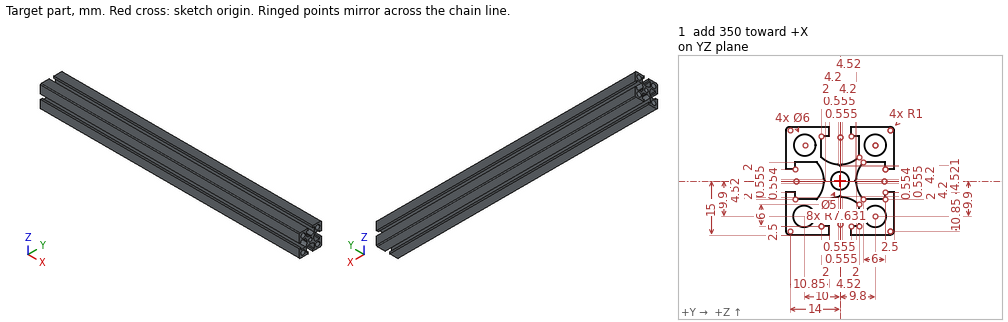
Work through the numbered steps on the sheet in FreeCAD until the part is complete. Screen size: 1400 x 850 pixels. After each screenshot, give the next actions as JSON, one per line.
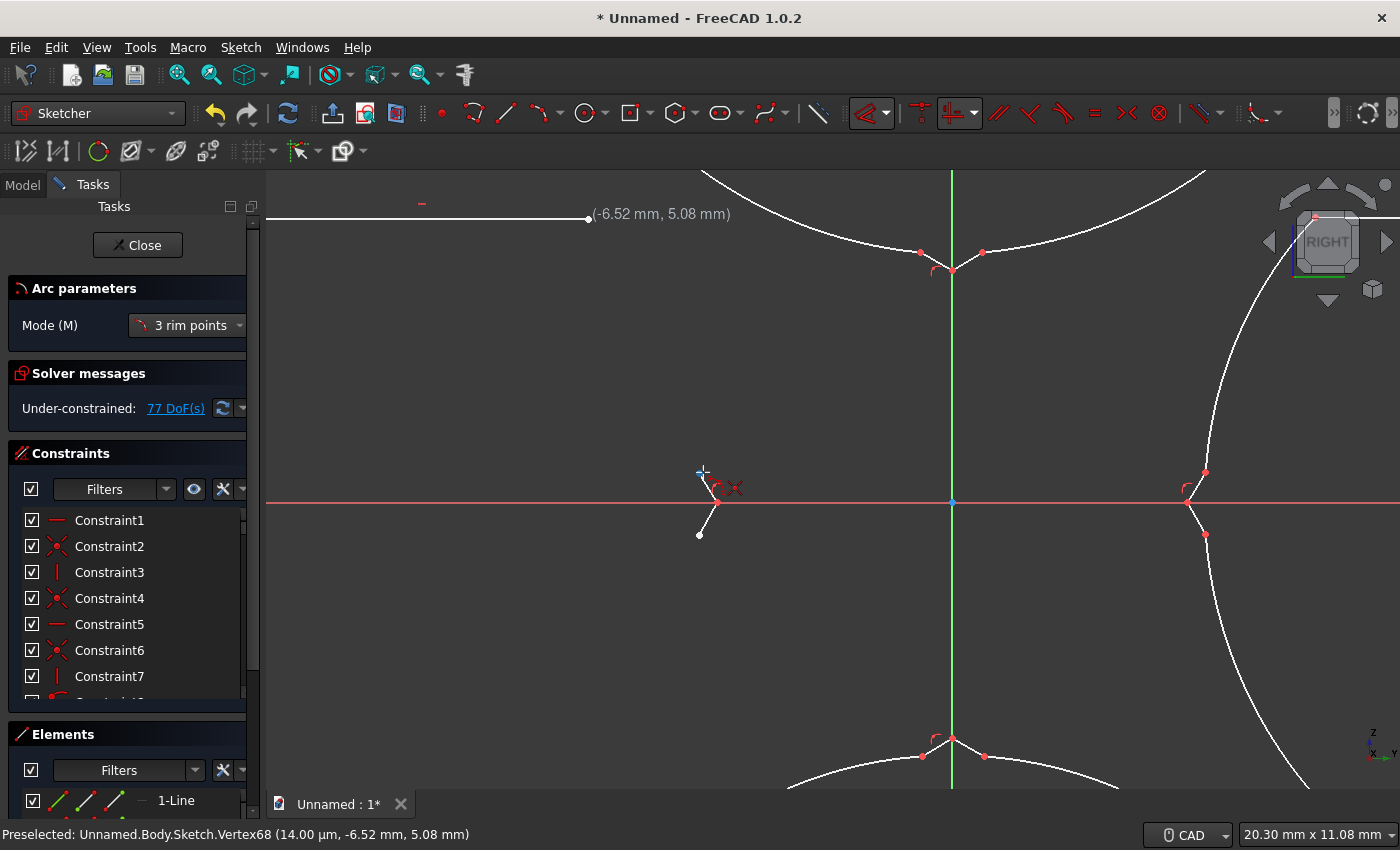
{"action": "left_click", "coordinate": [699, 473]}
{"action": "left_click", "coordinate": [666, 334]}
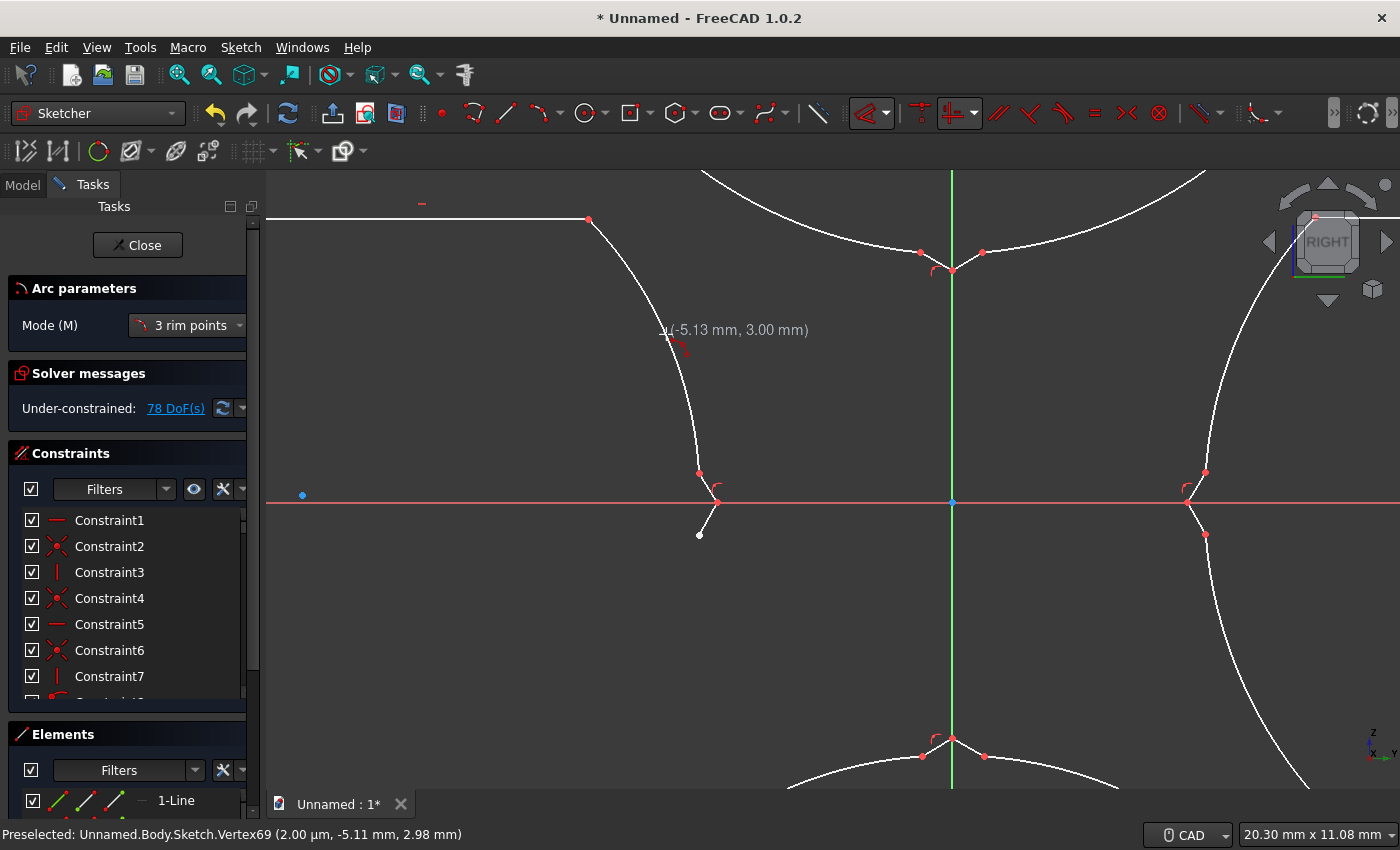
{"action": "left_click", "coordinate": [699, 535]}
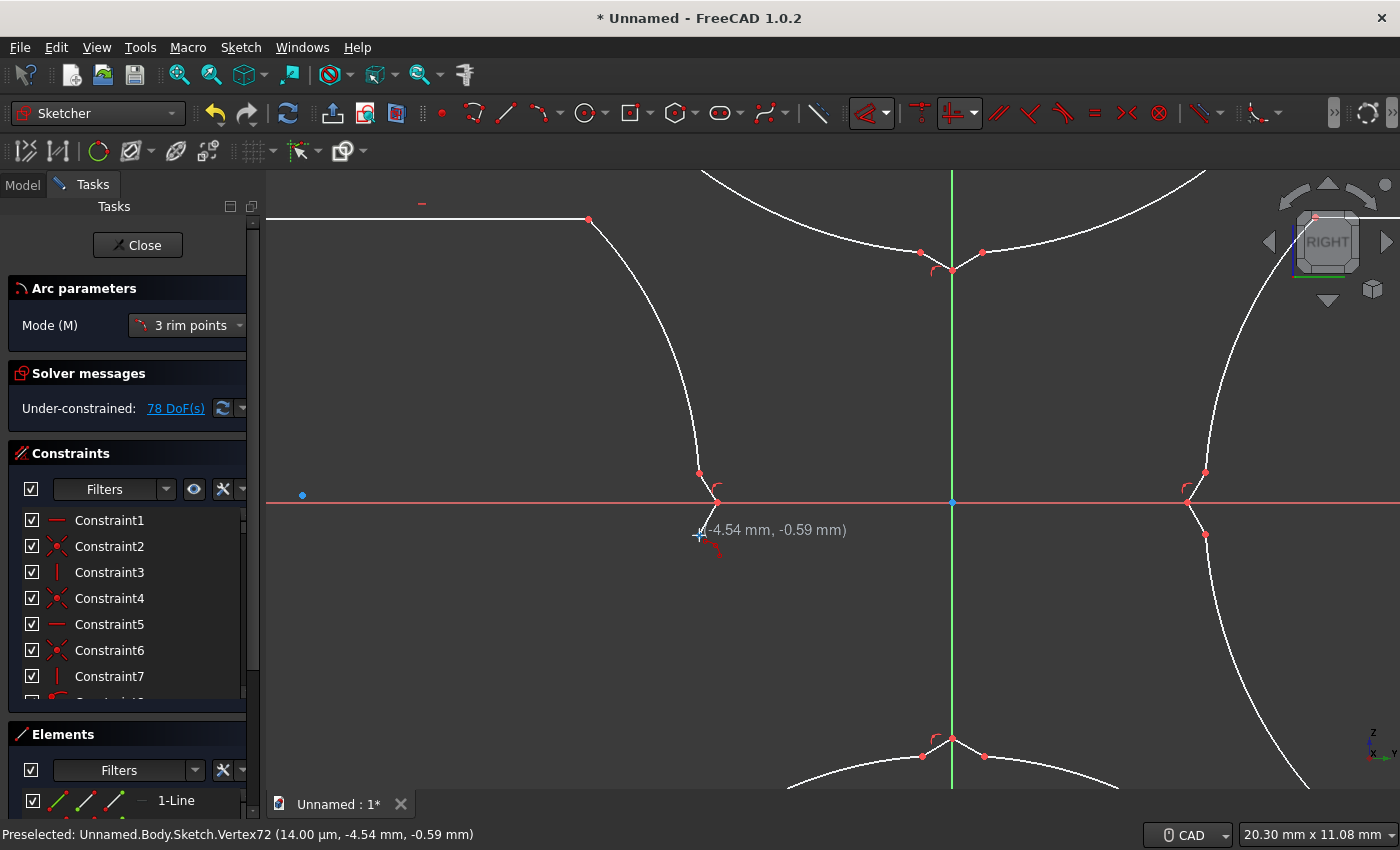
{"action": "scroll", "coordinate": [703, 472], "scroll_direction": "down", "scroll_amount": 7}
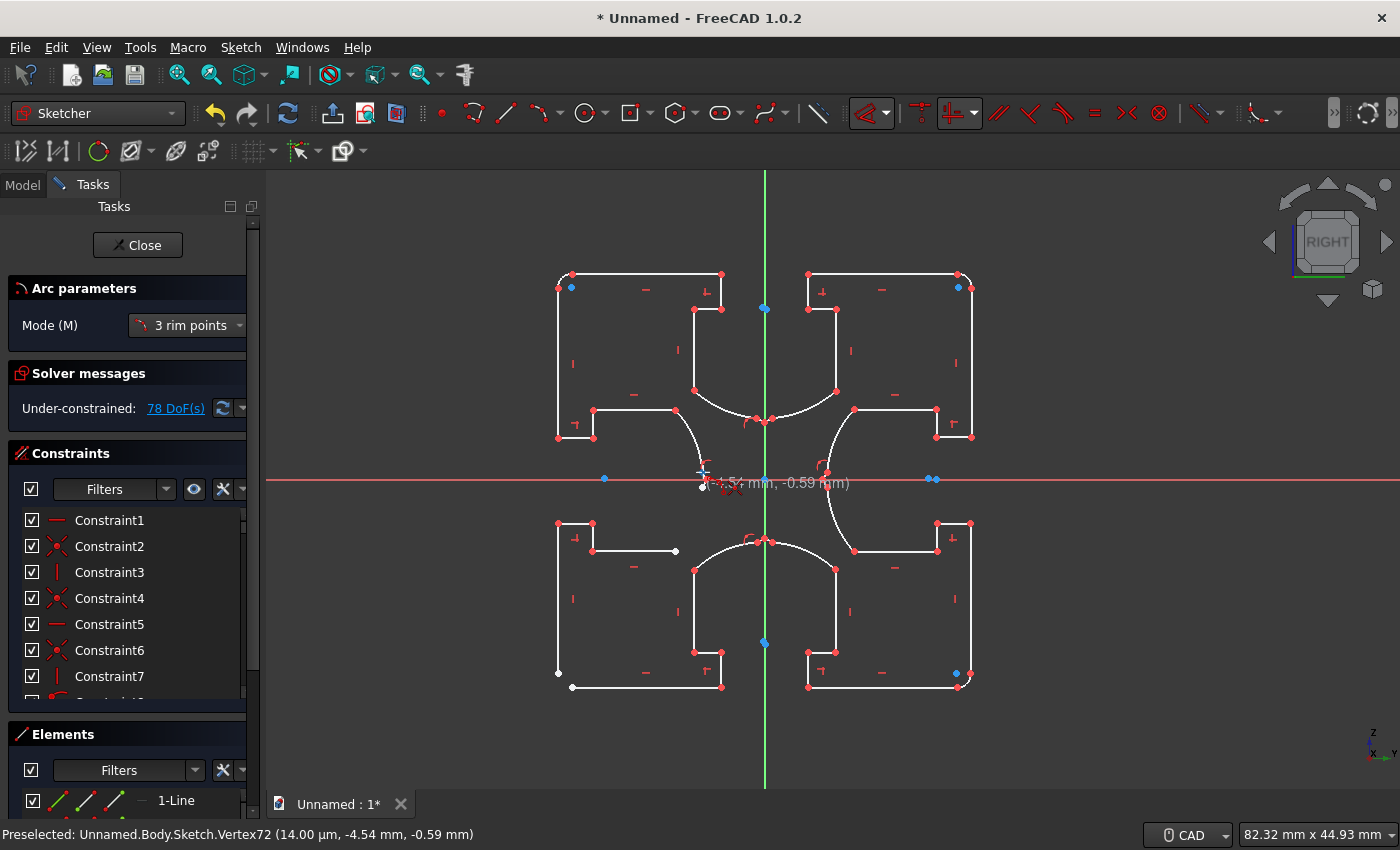
{"action": "left_click", "coordinate": [675, 551]}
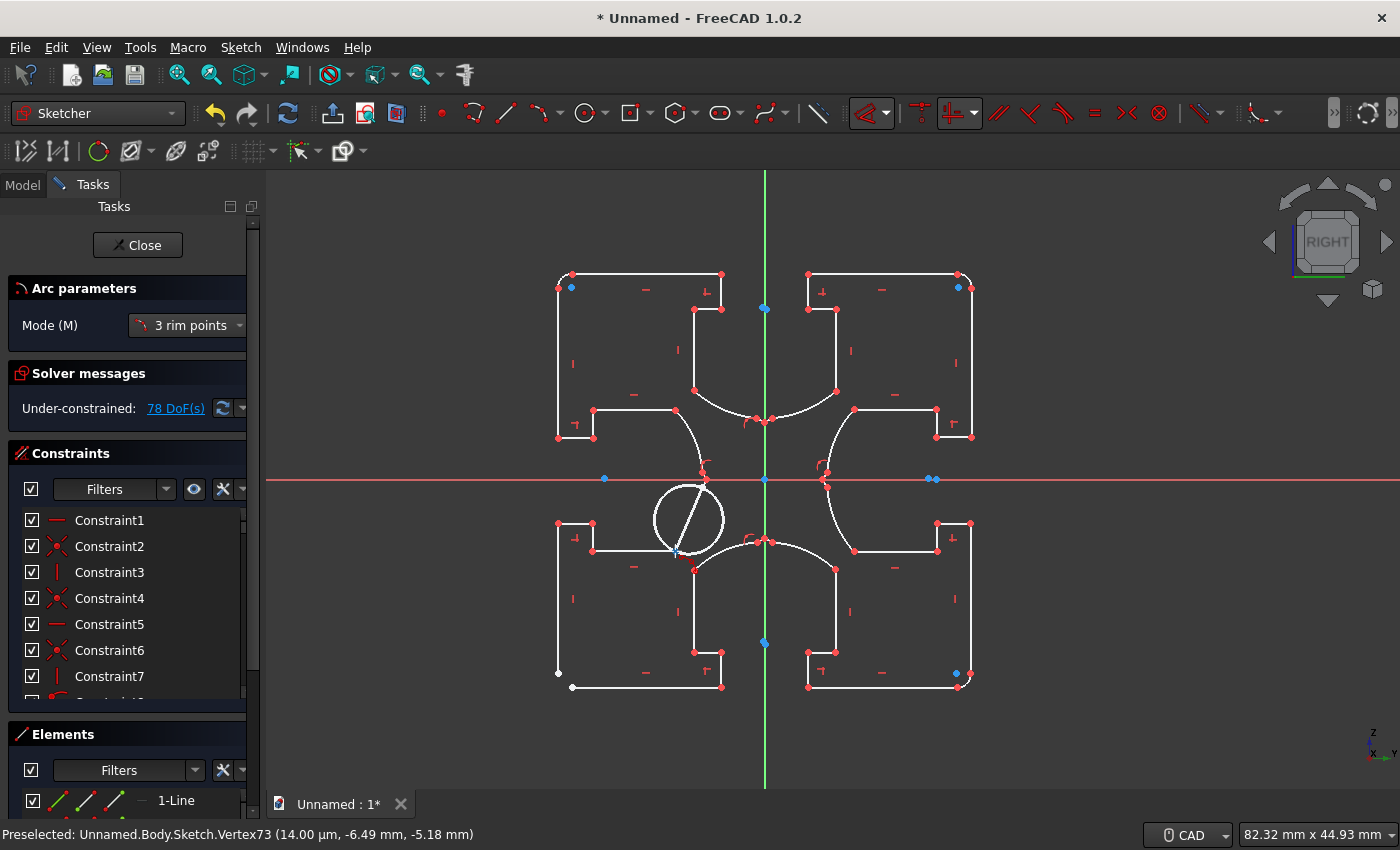
{"action": "scroll", "coordinate": [694, 522], "scroll_direction": "up", "scroll_amount": 6}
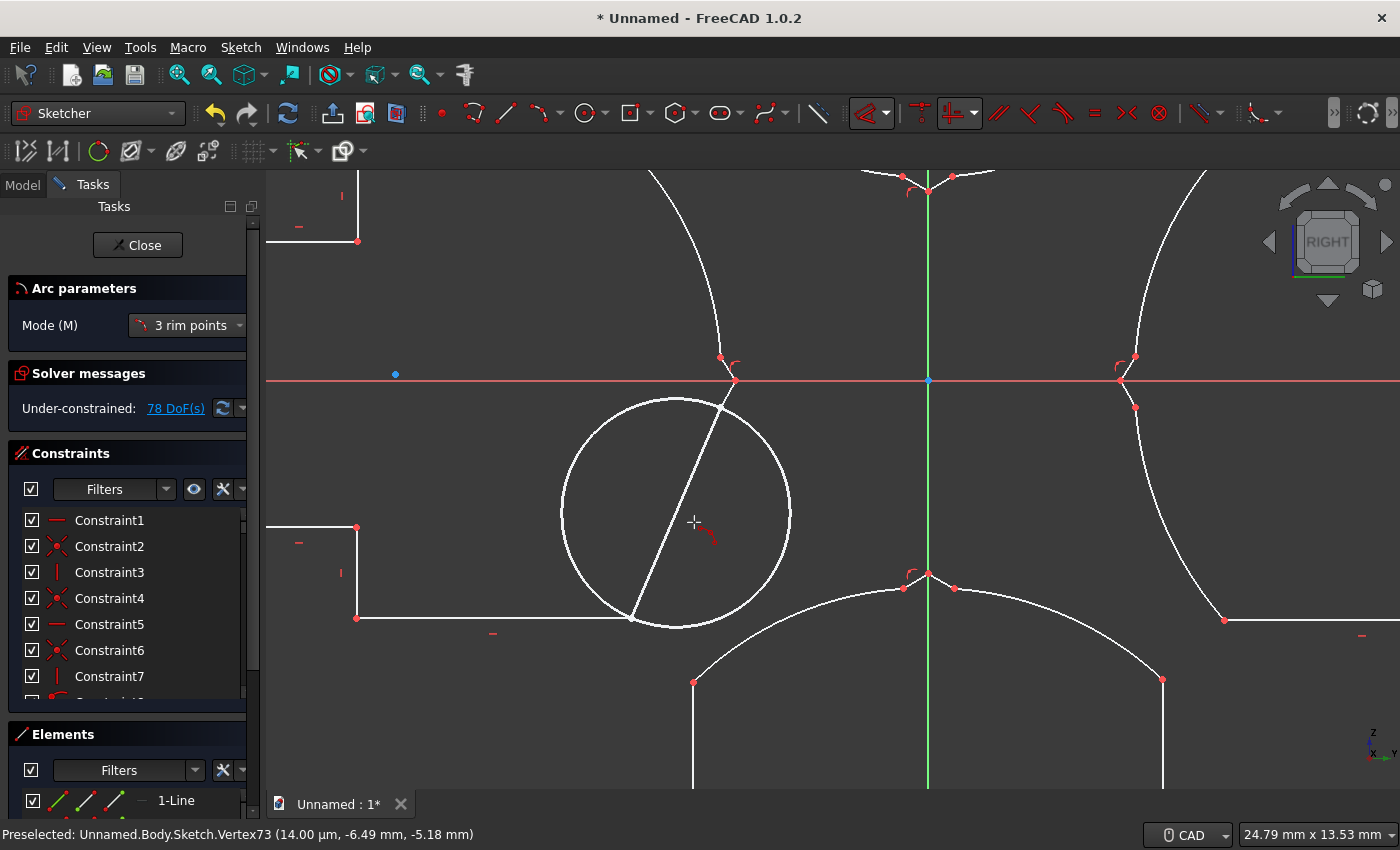
{"action": "left_click", "coordinate": [694, 519]}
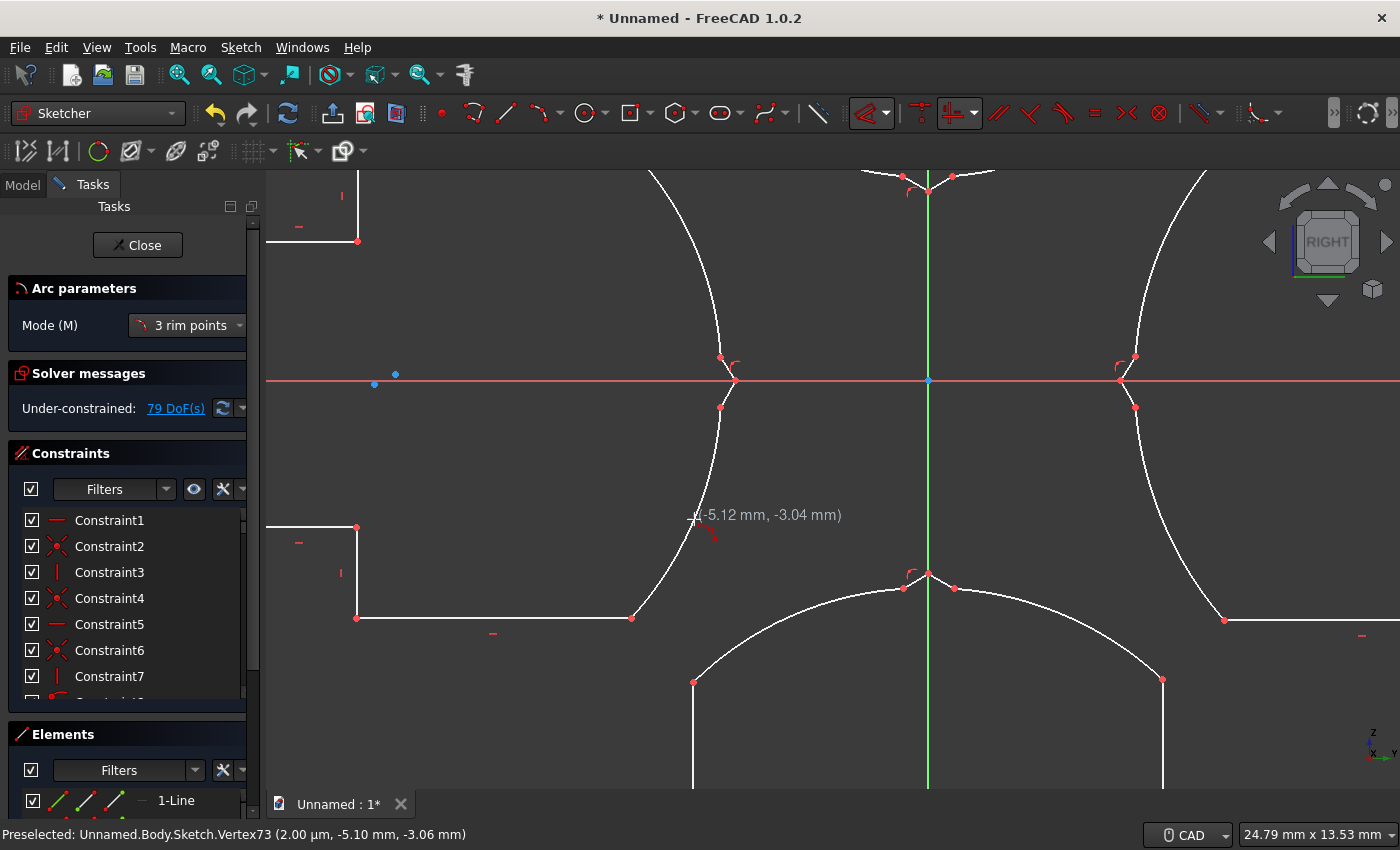
{"action": "scroll", "coordinate": [694, 522], "scroll_direction": "down", "scroll_amount": 6}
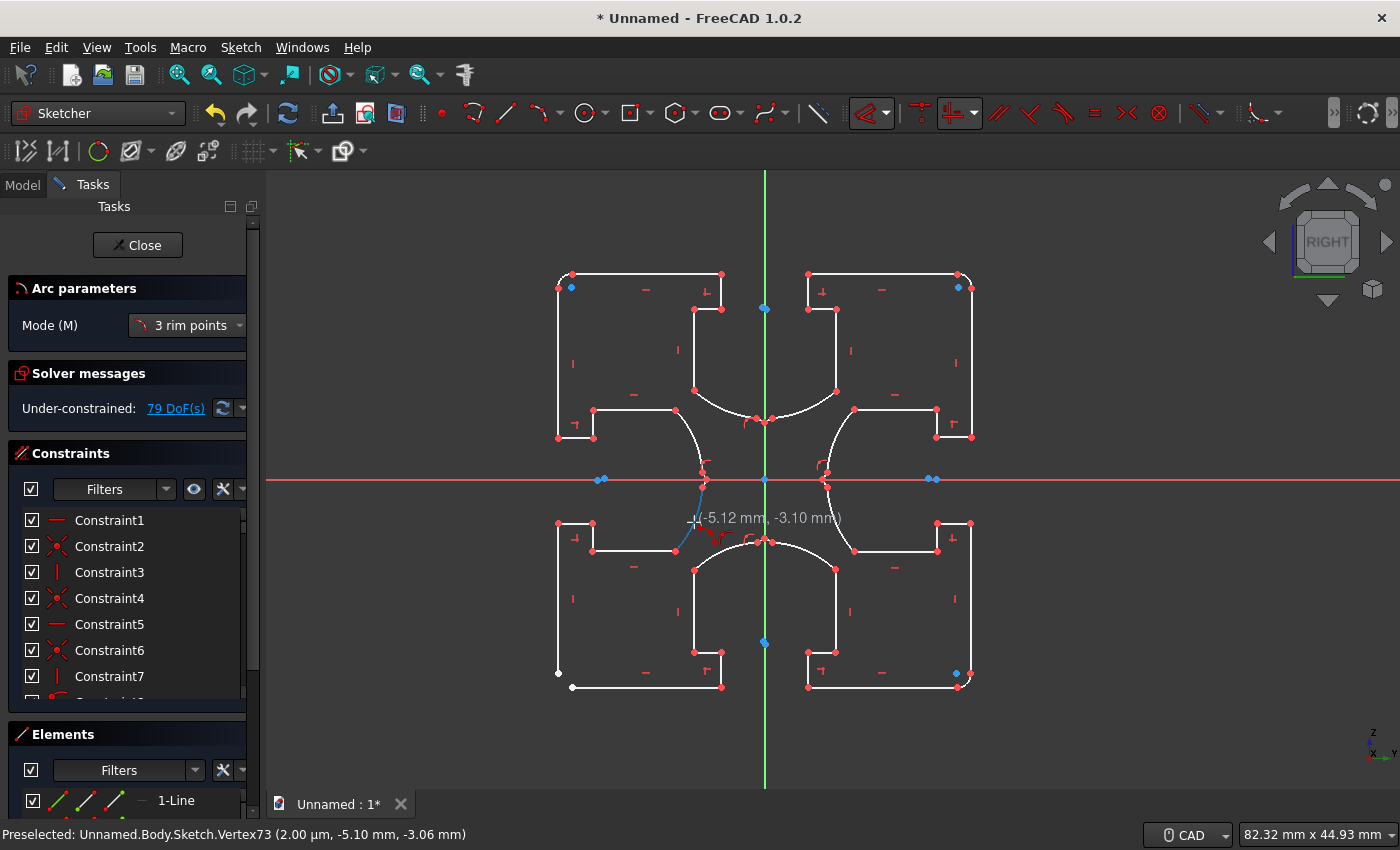
{"action": "left_click", "coordinate": [558, 674]}
{"action": "left_click", "coordinate": [572, 688]}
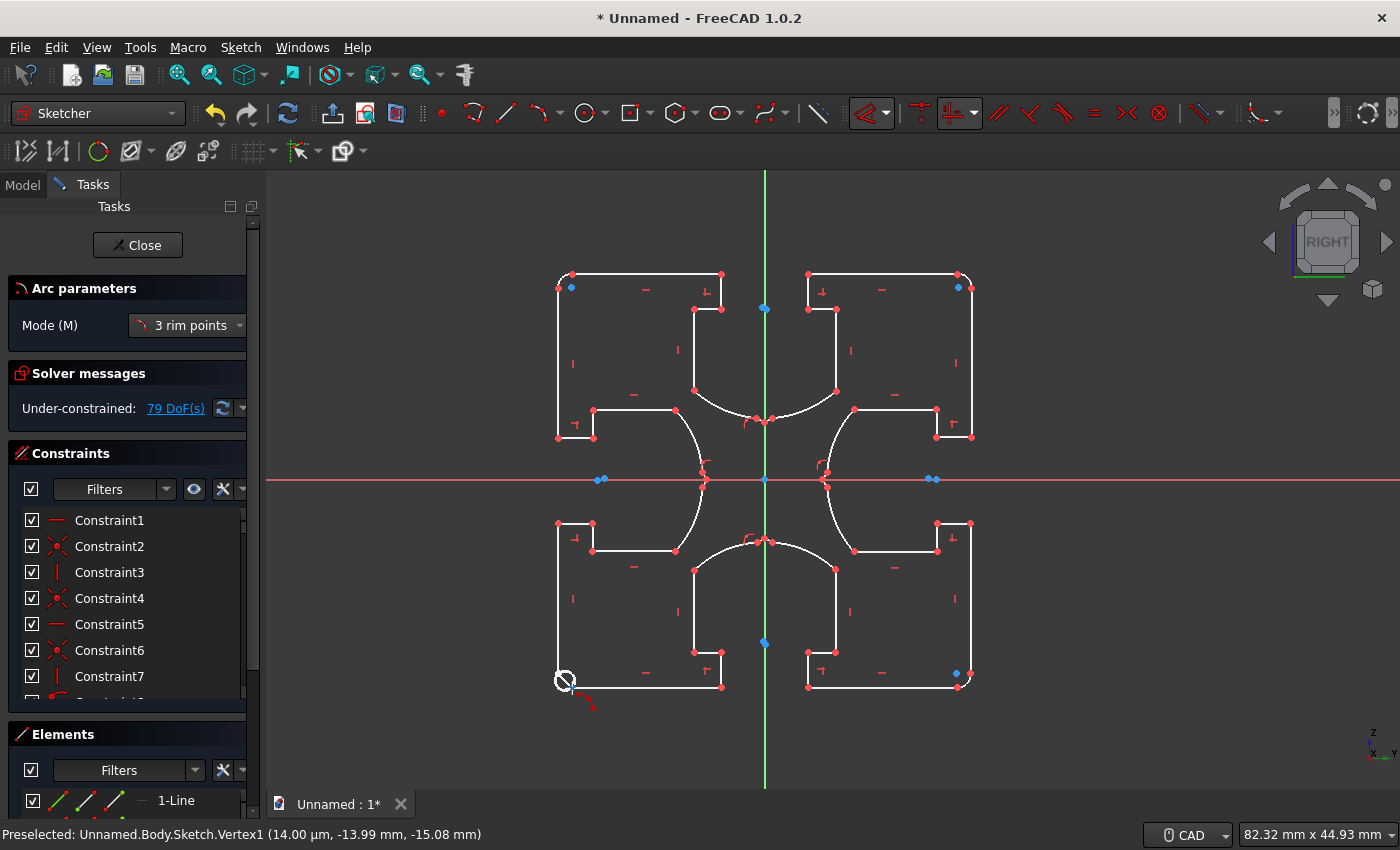
{"action": "scroll", "coordinate": [562, 683], "scroll_direction": "up", "scroll_amount": 7}